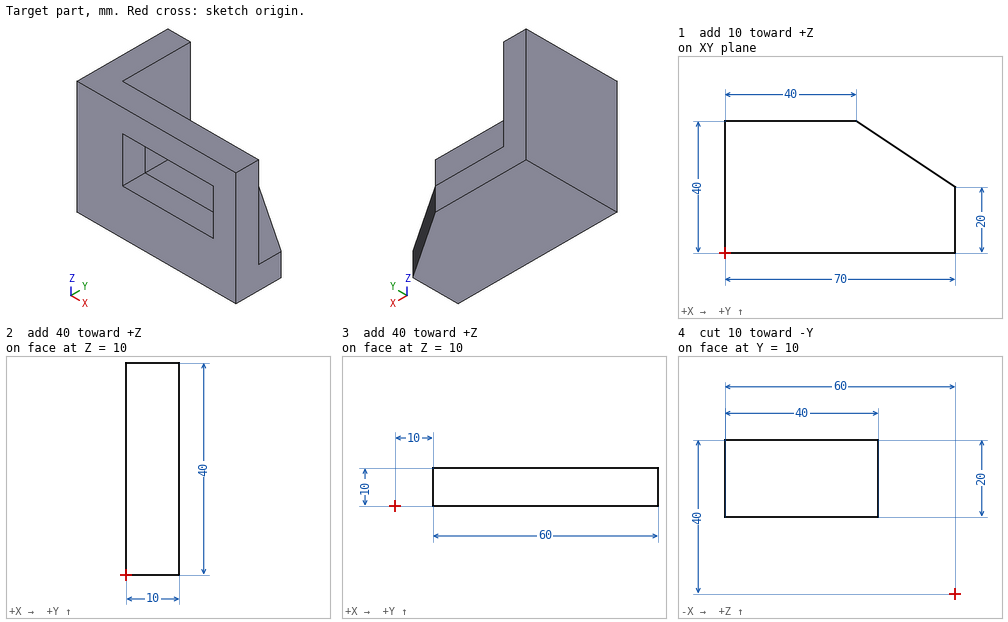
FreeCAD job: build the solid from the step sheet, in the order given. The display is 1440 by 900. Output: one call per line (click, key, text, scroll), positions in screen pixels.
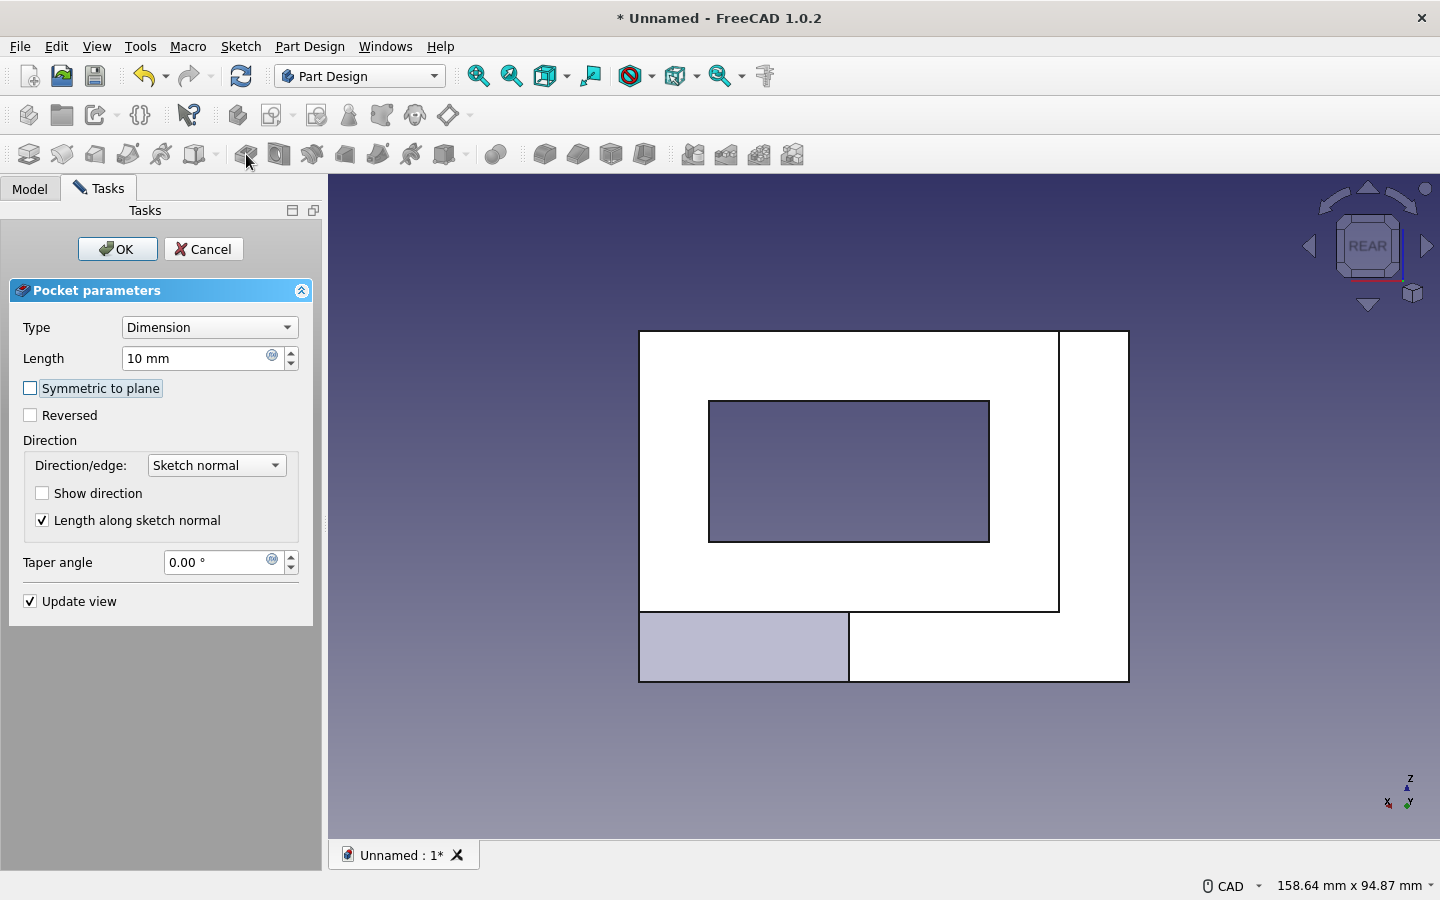
click(118, 249)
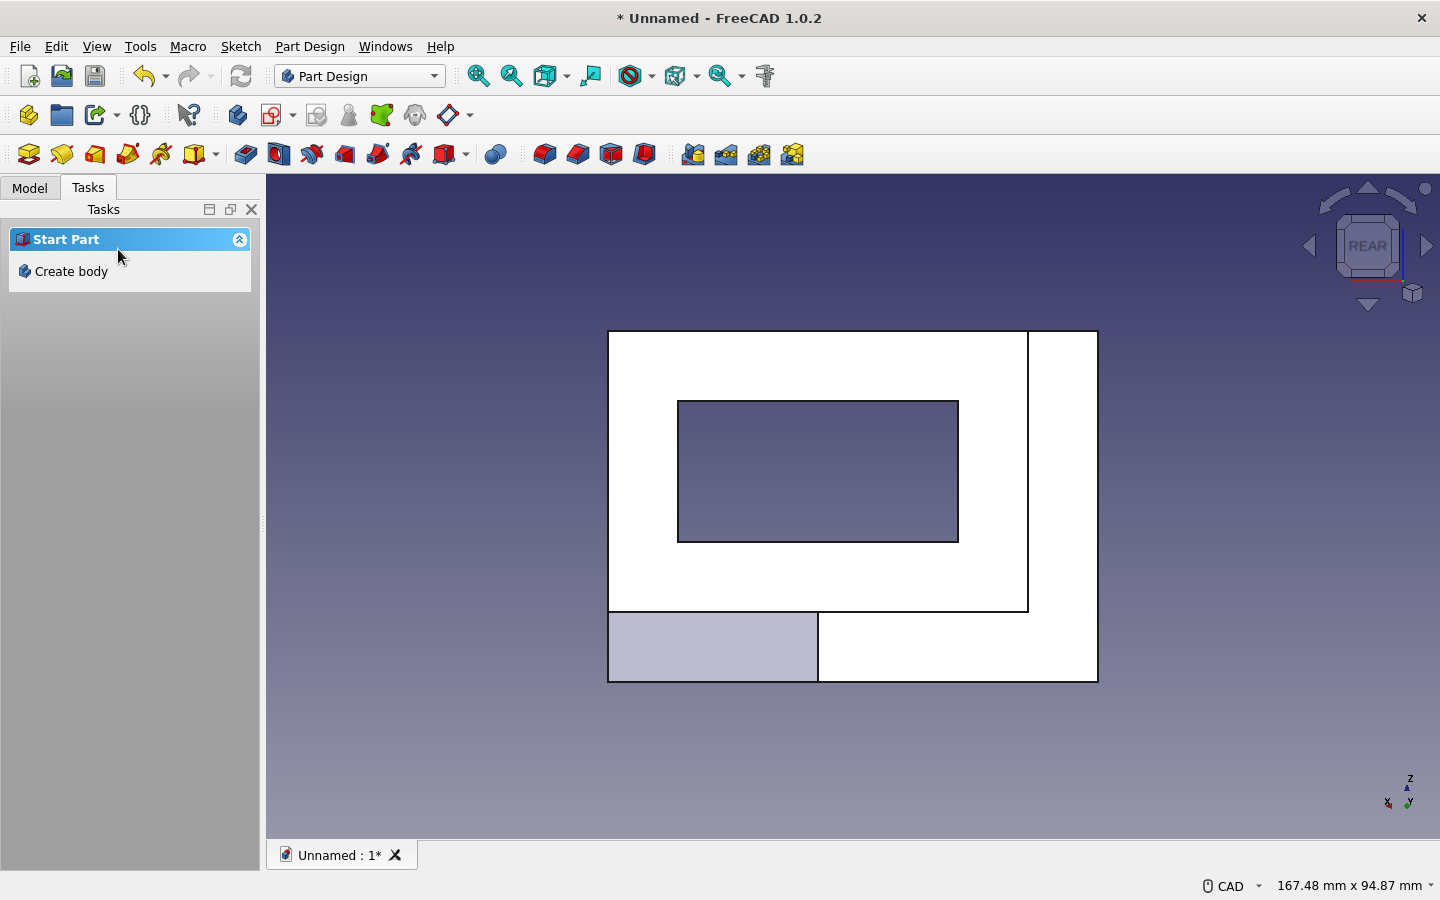
key(0)